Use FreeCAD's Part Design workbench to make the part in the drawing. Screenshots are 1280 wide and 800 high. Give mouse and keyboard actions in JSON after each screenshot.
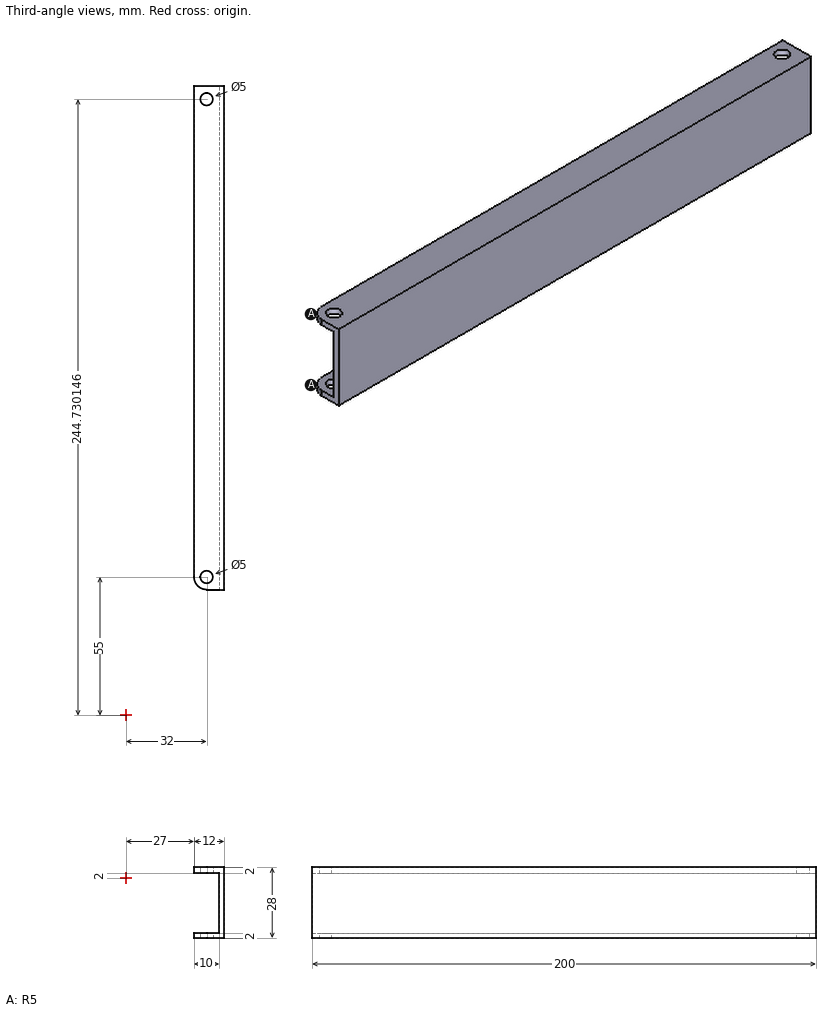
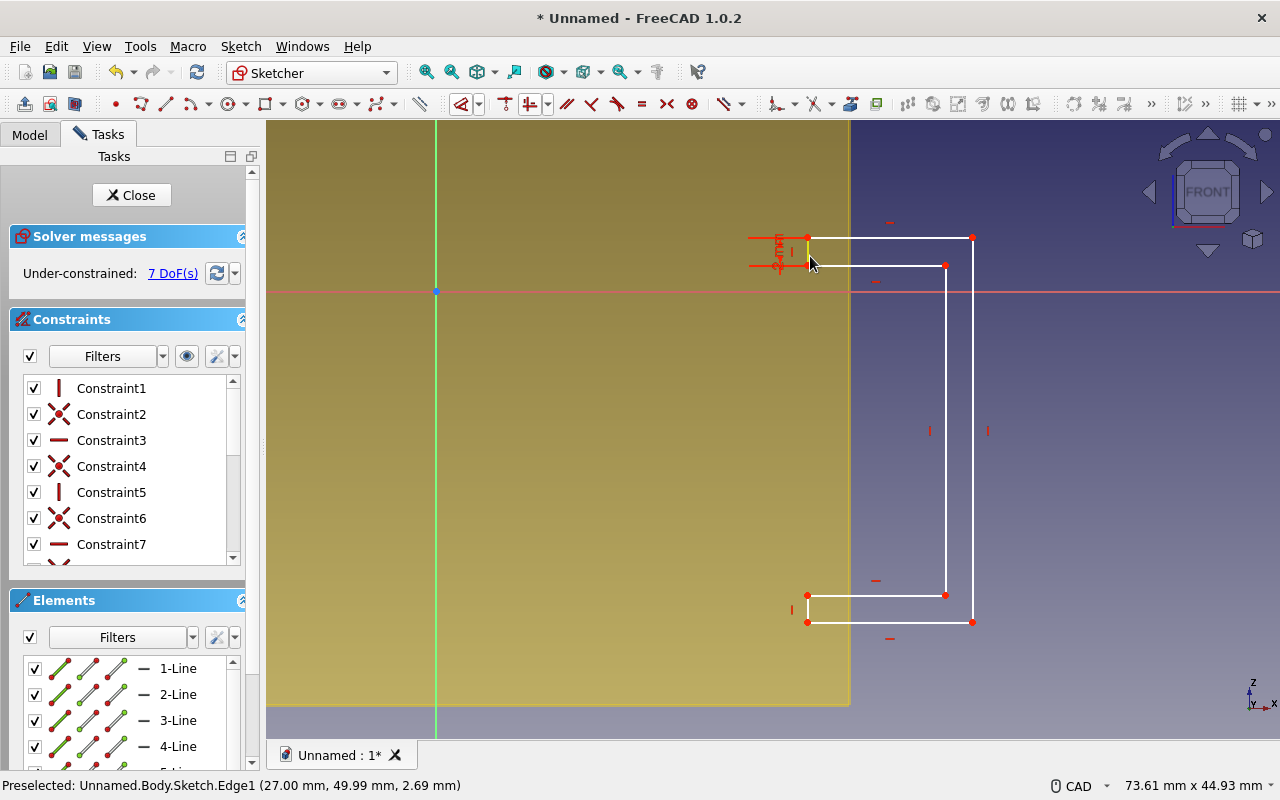
{"action": "scroll", "coordinate": [808, 615], "scroll_direction": "up", "scroll_amount": 3}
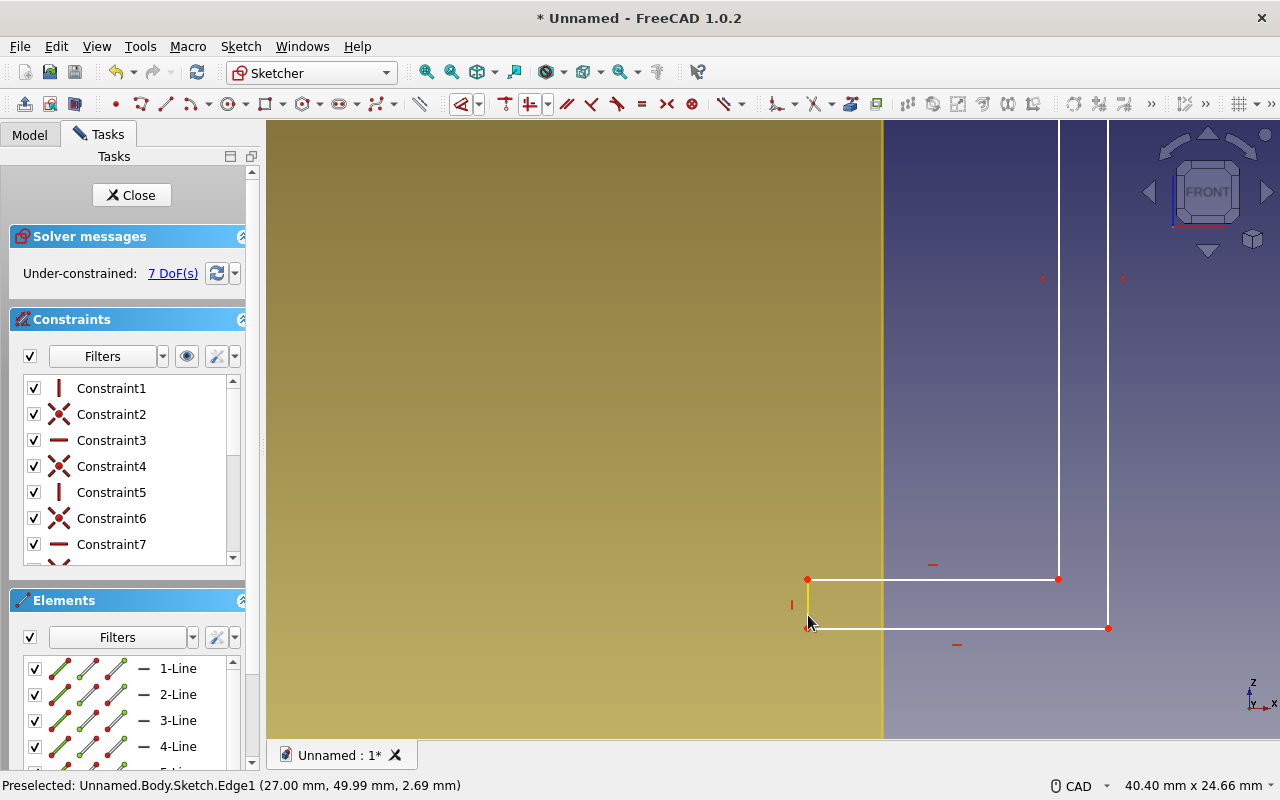
{"action": "left_click", "coordinate": [808, 614]}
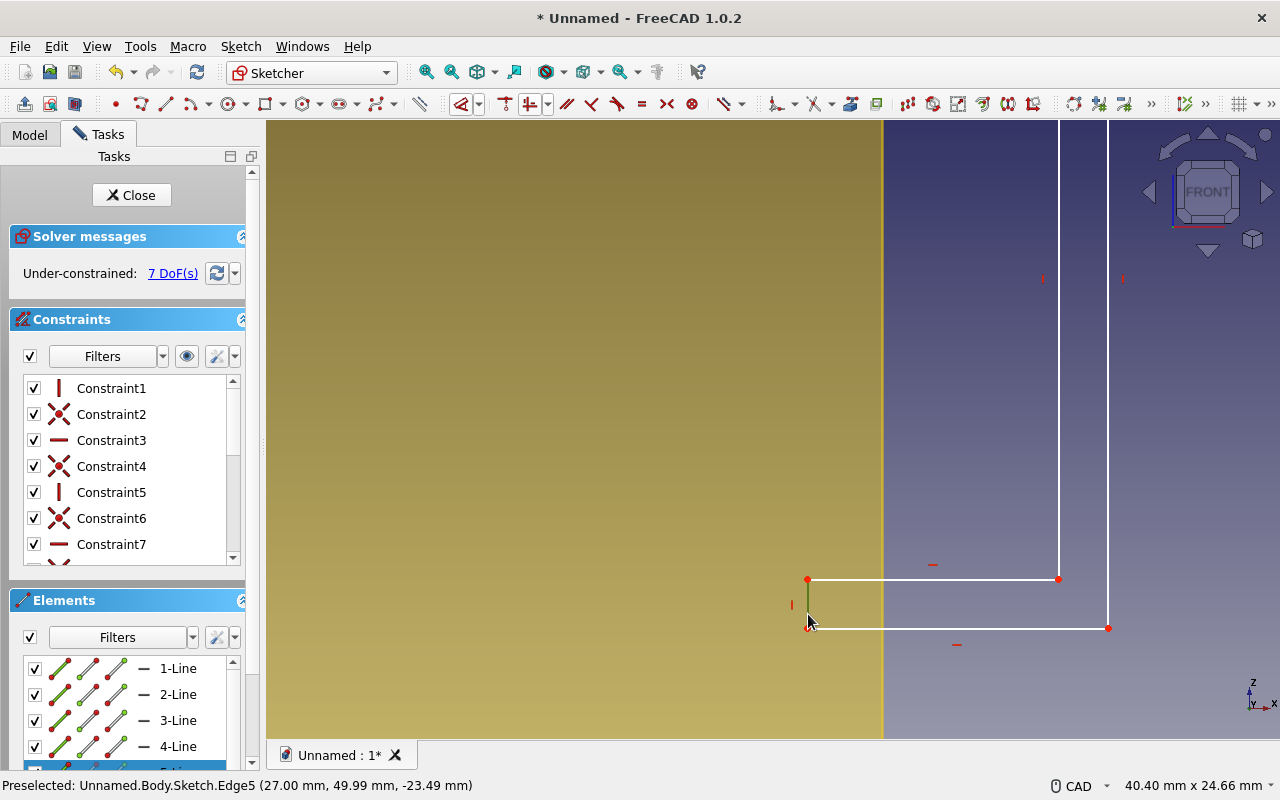
{"action": "key", "text": "i"}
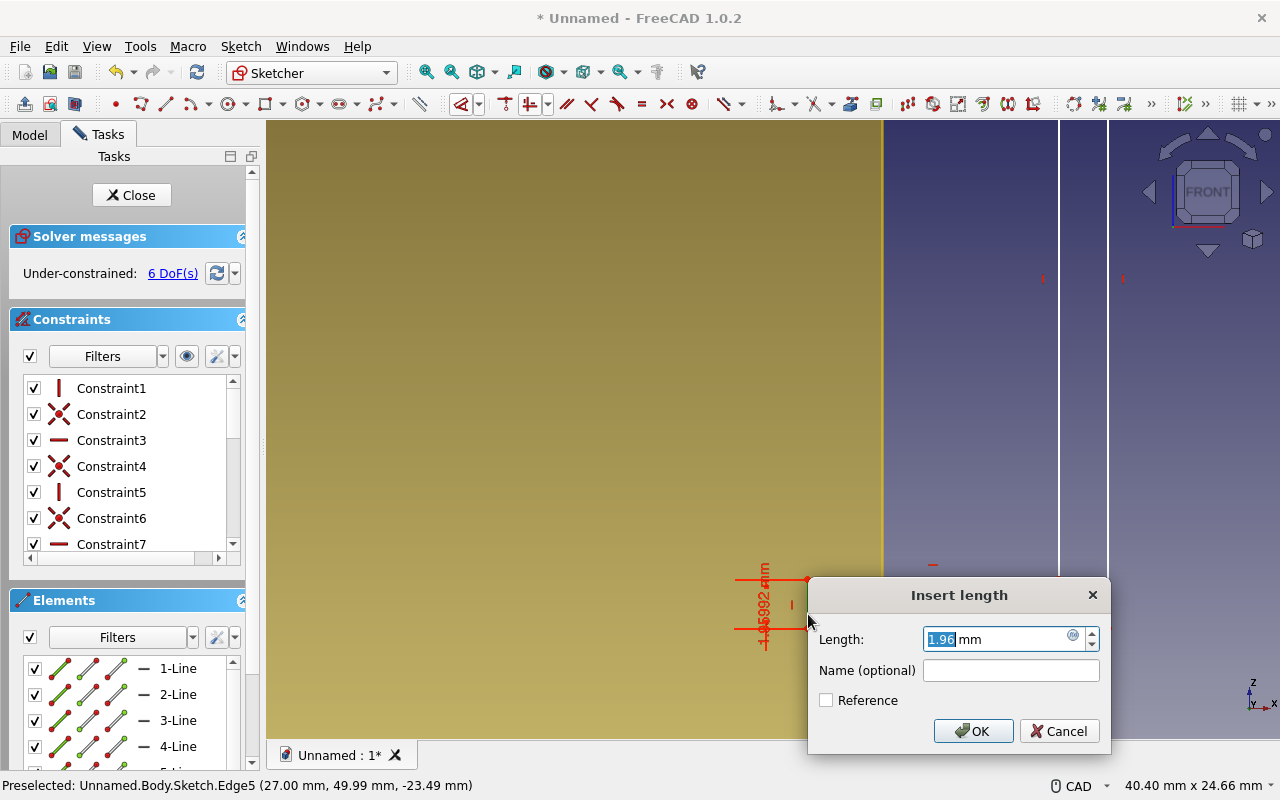
{"action": "type", "text": "2"}
{"action": "key", "text": "Return"}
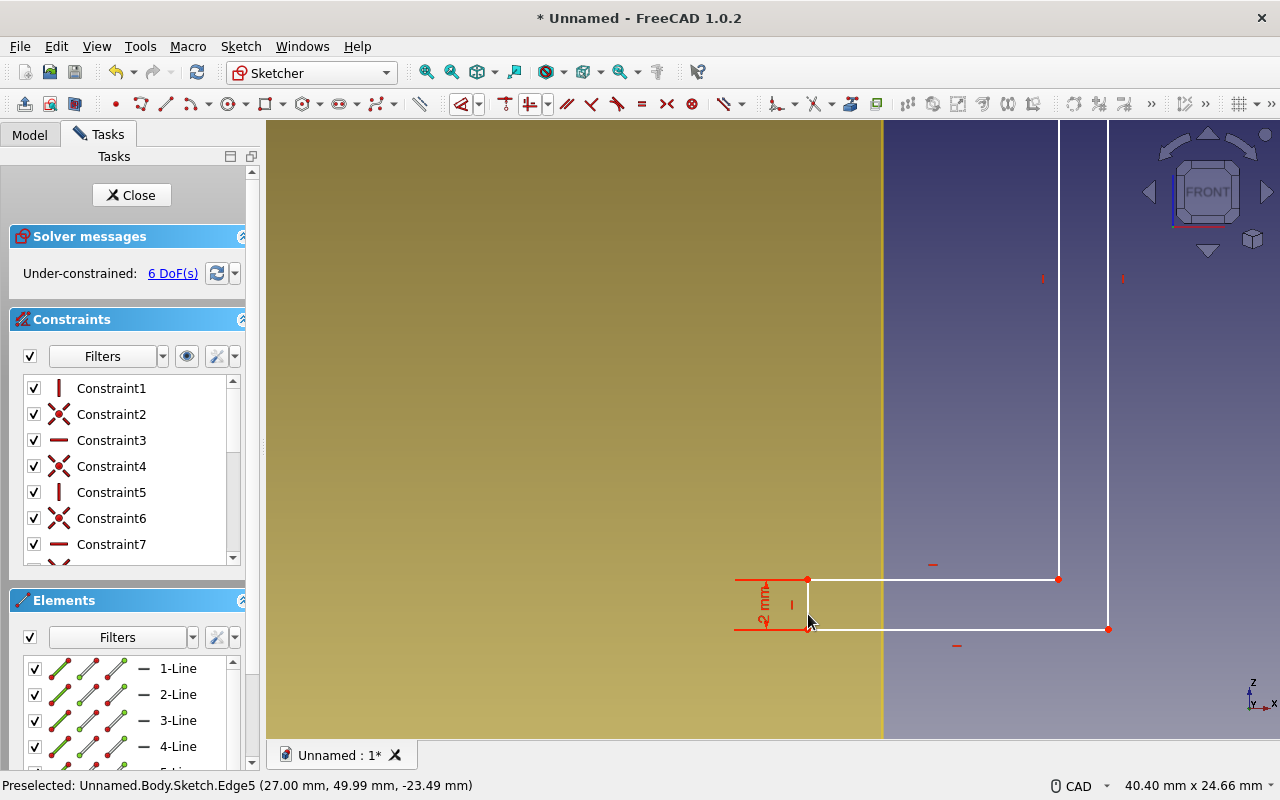
{"action": "scroll", "coordinate": [808, 616], "scroll_direction": "down", "scroll_amount": 3}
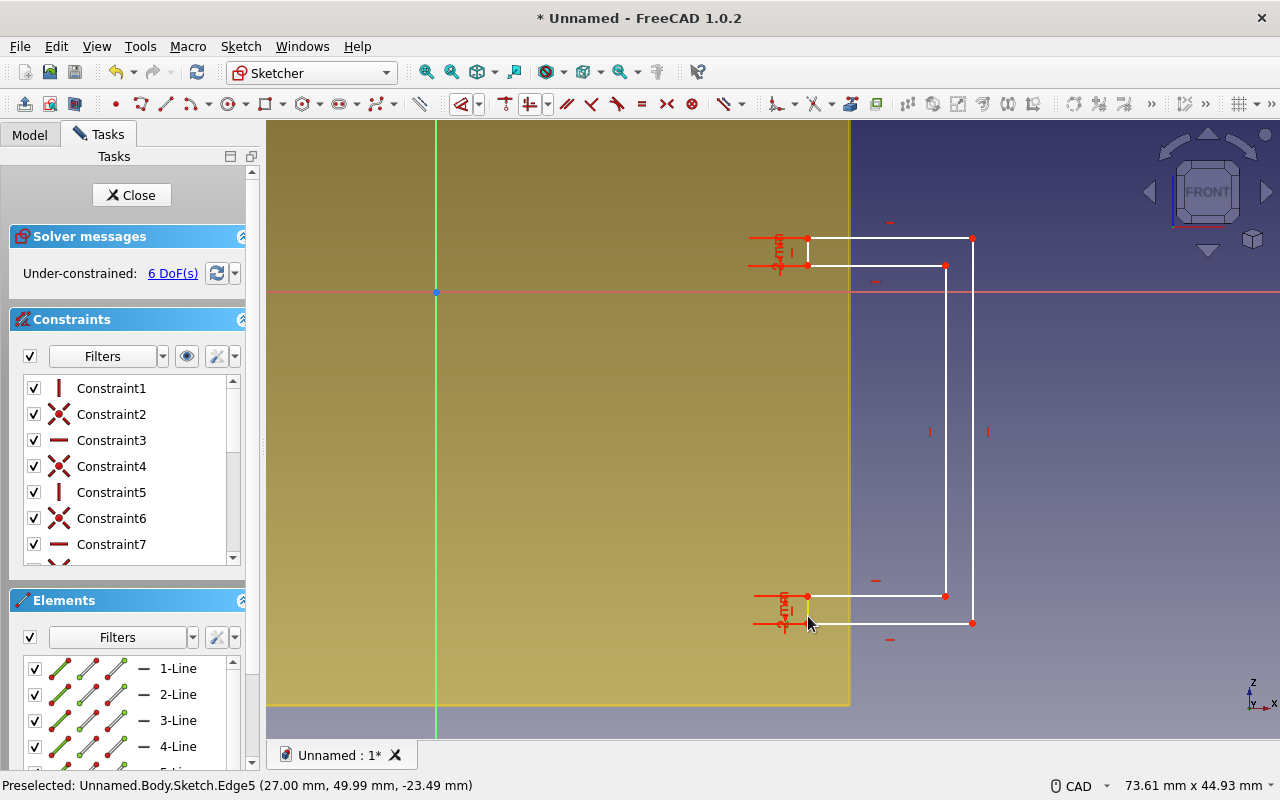
{"action": "left_click", "coordinate": [857, 238]}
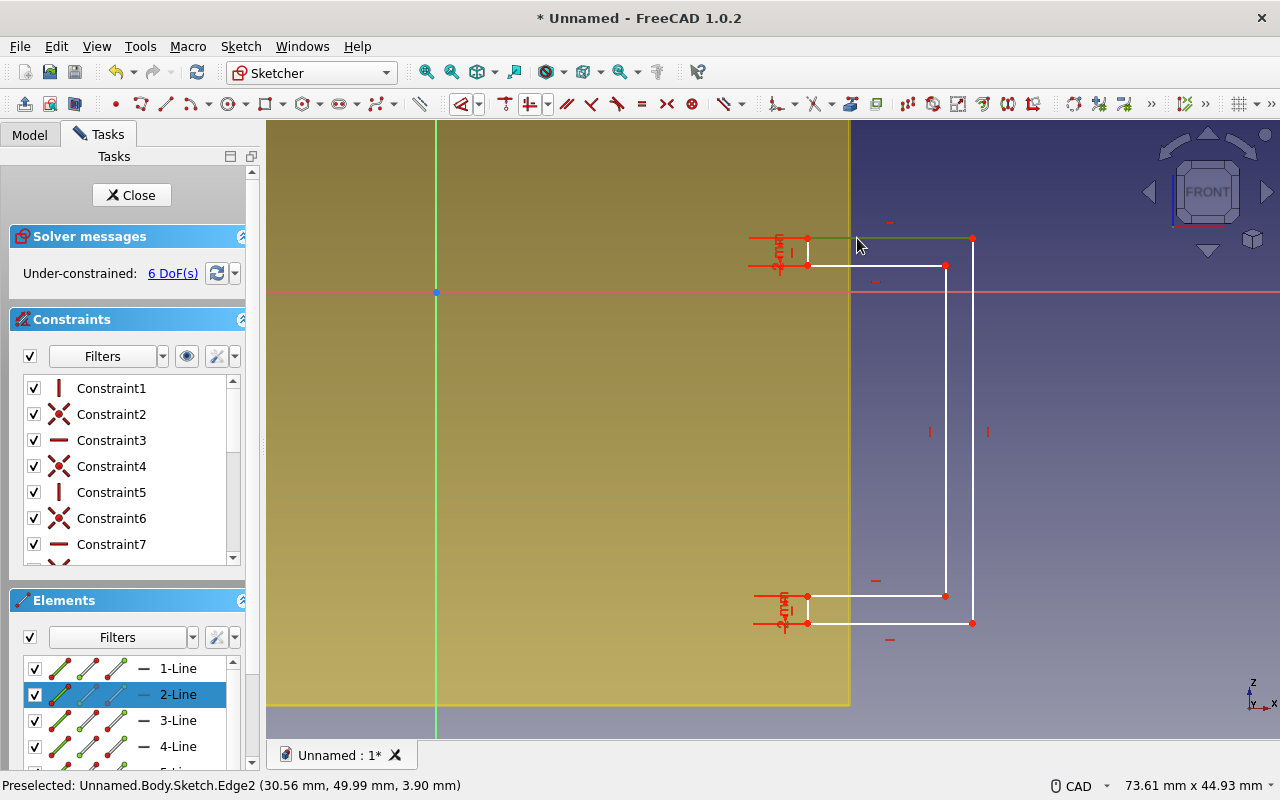
{"action": "left_click", "coordinate": [478, 104]}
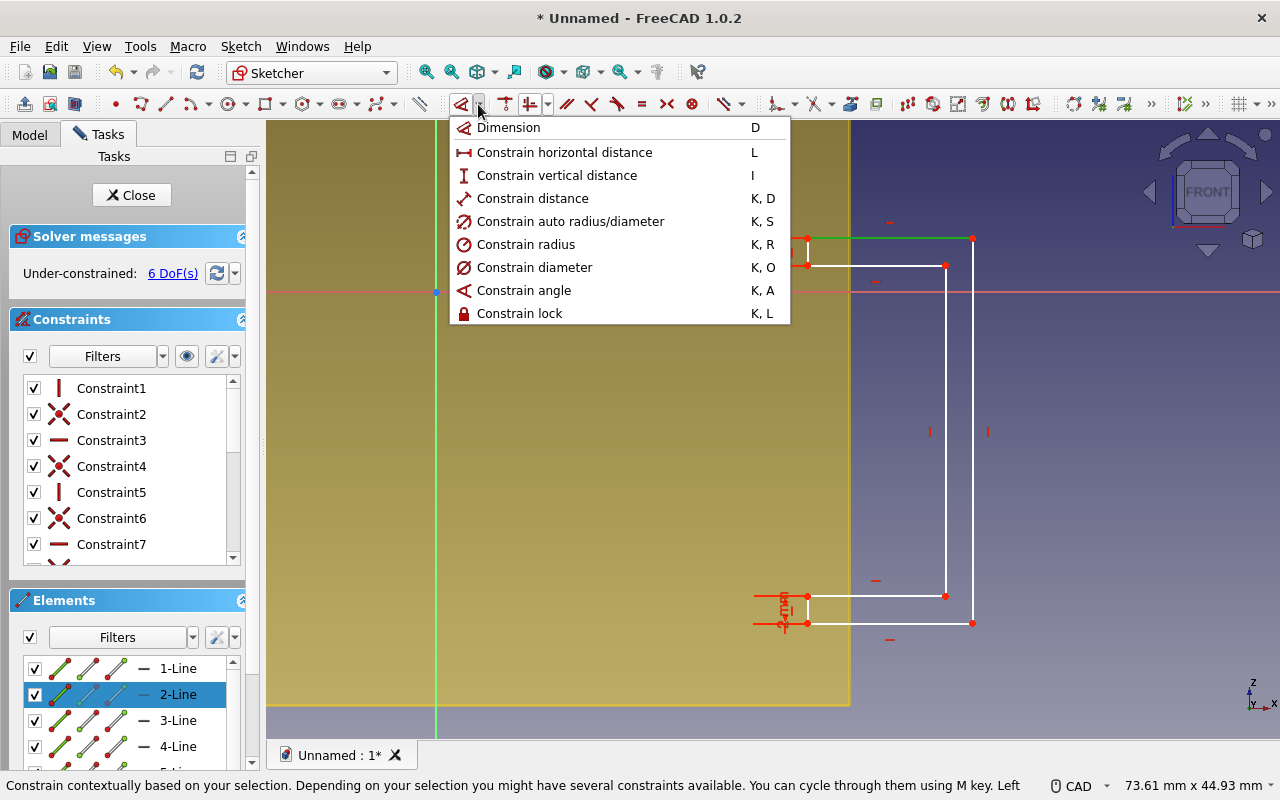
{"action": "left_click", "coordinate": [620, 152]}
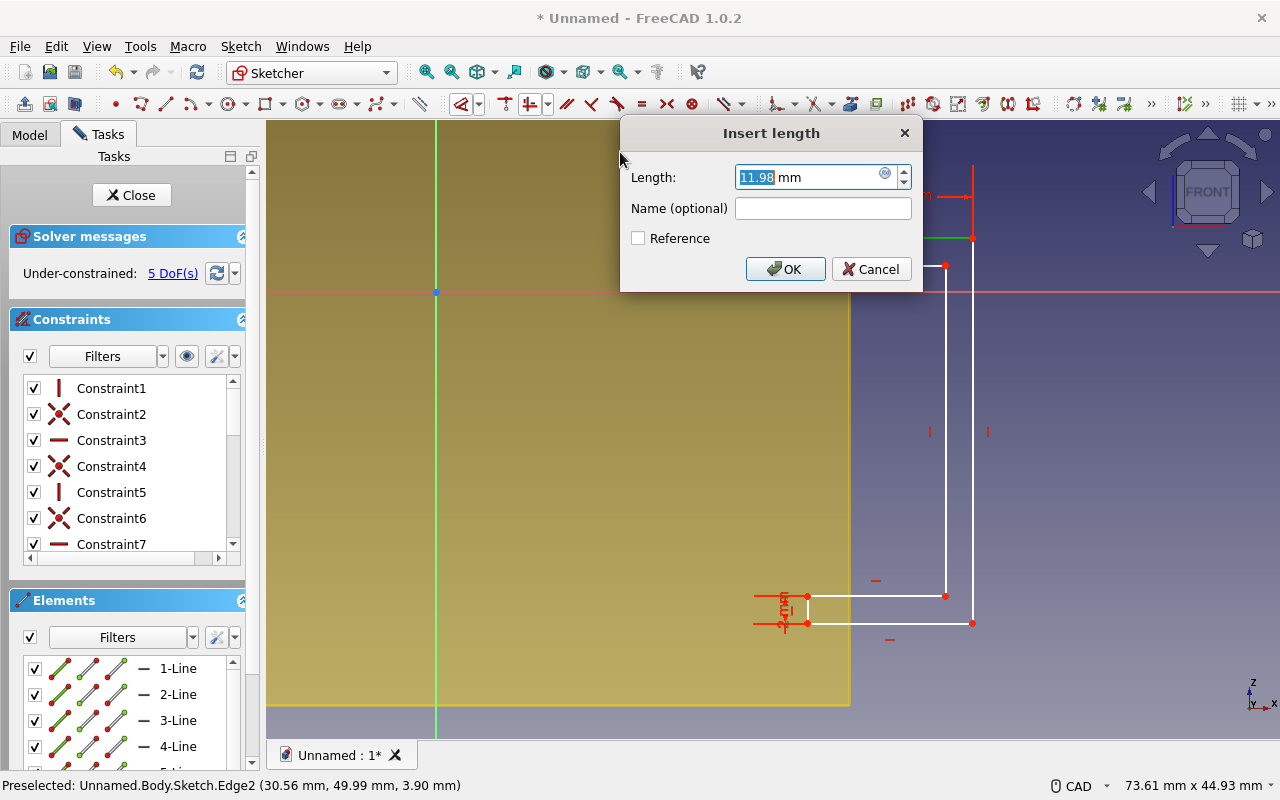
{"action": "type", "text": "12"}
{"action": "key", "text": "Return"}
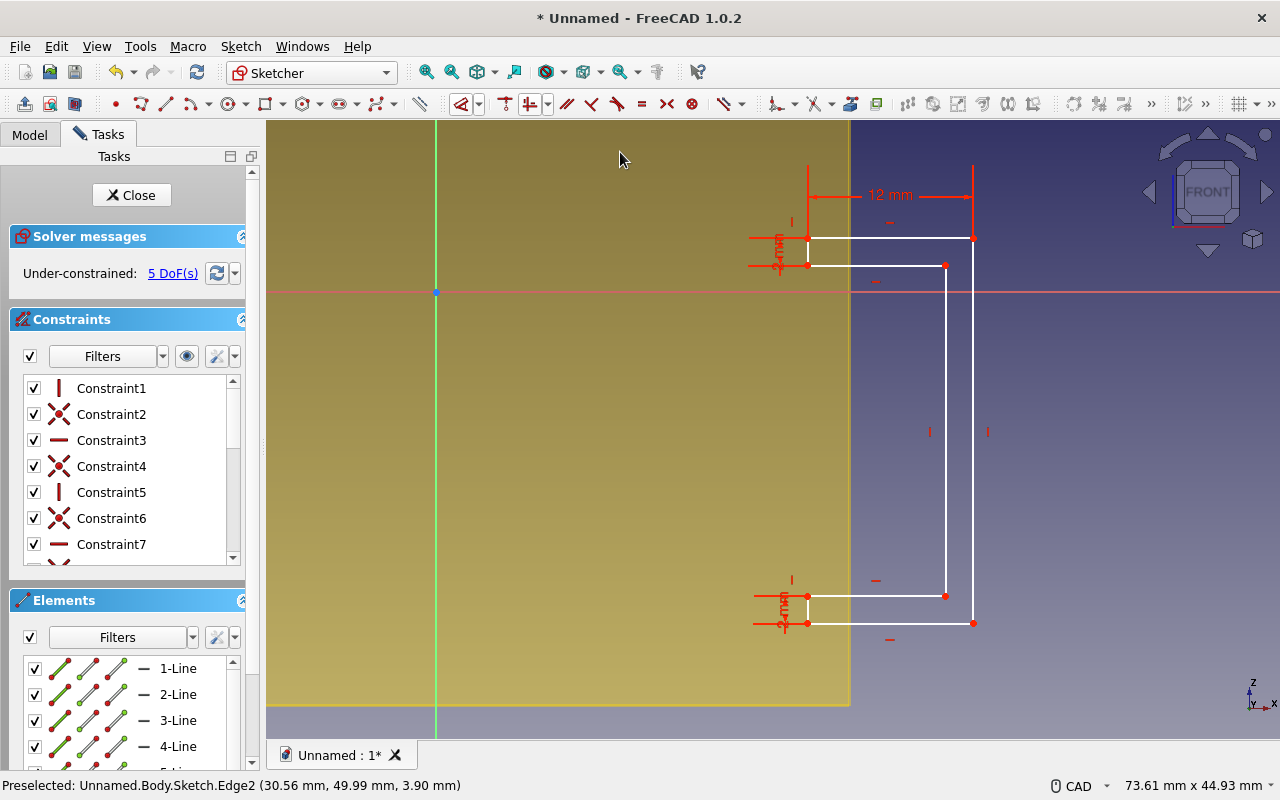
{"action": "left_click", "coordinate": [973, 354]}